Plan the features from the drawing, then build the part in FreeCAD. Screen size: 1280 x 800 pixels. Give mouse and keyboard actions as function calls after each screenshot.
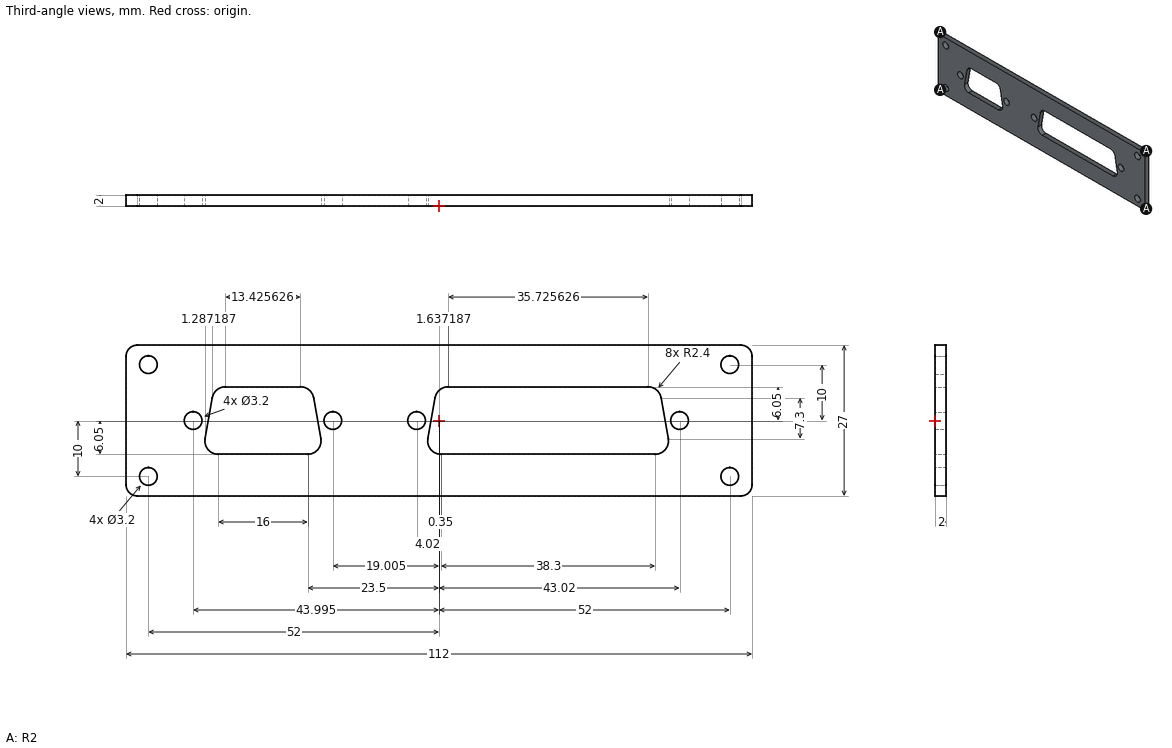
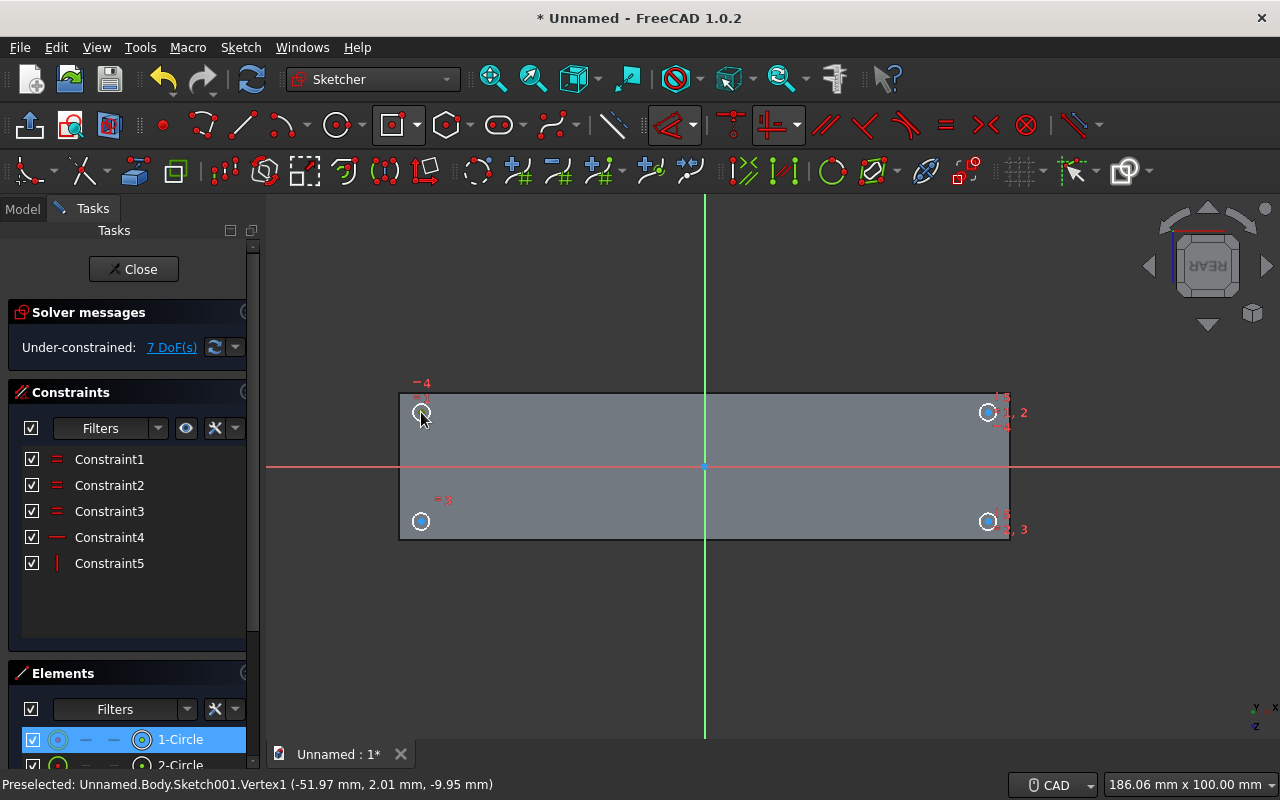
click(421, 522)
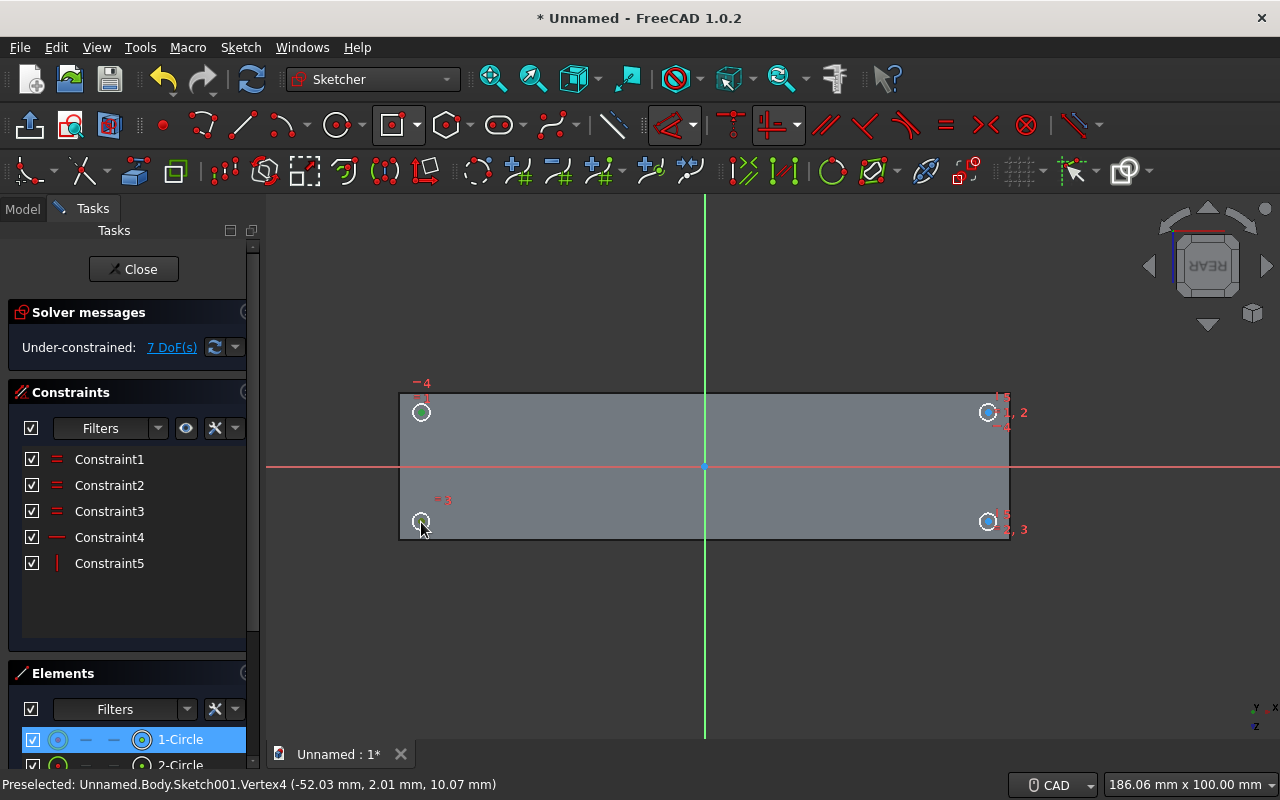
key(v)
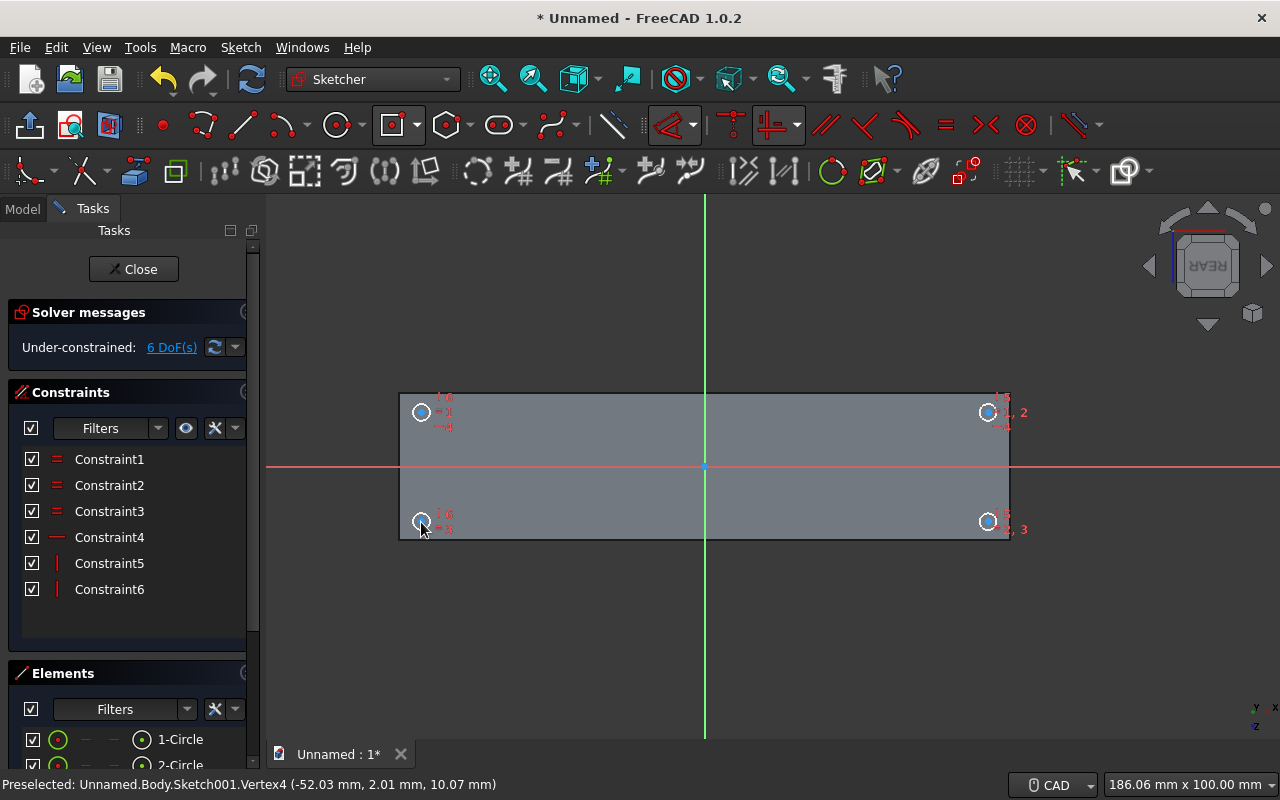
click(988, 522)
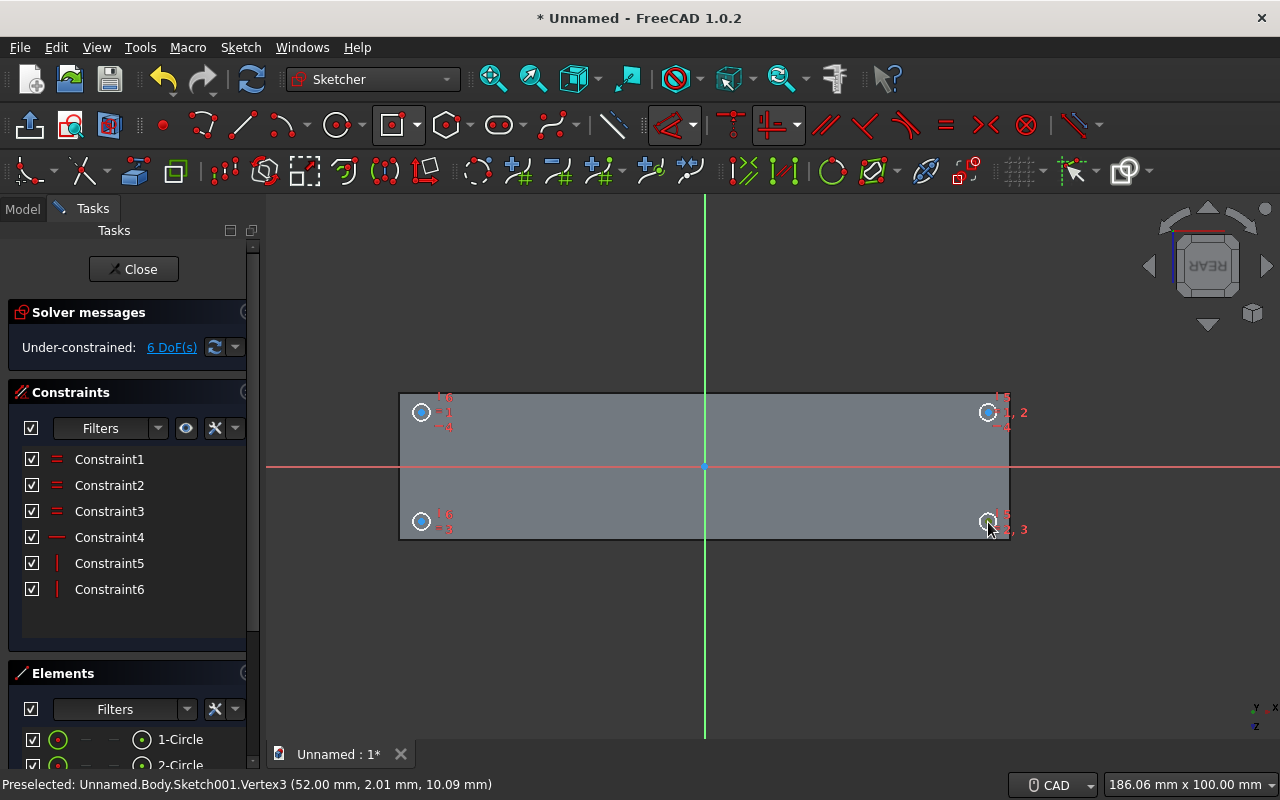
click(421, 522)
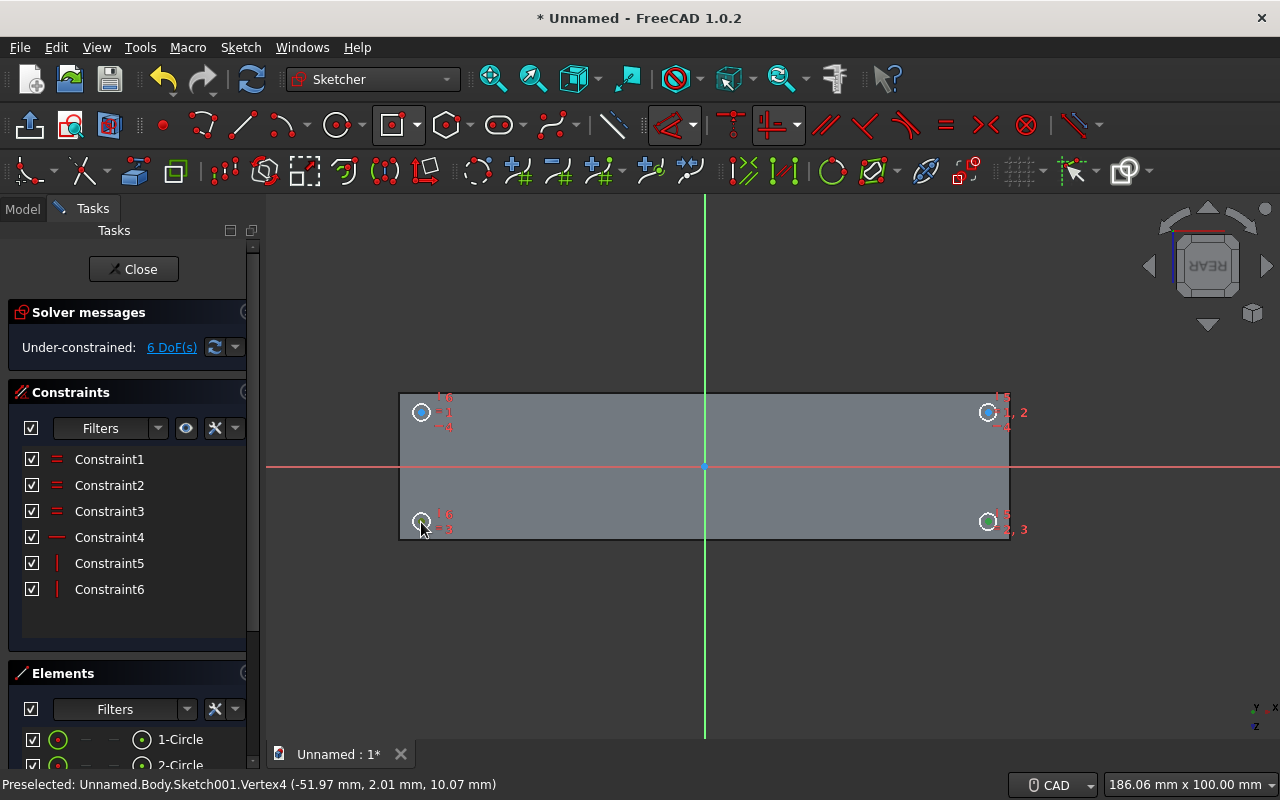
click(800, 126)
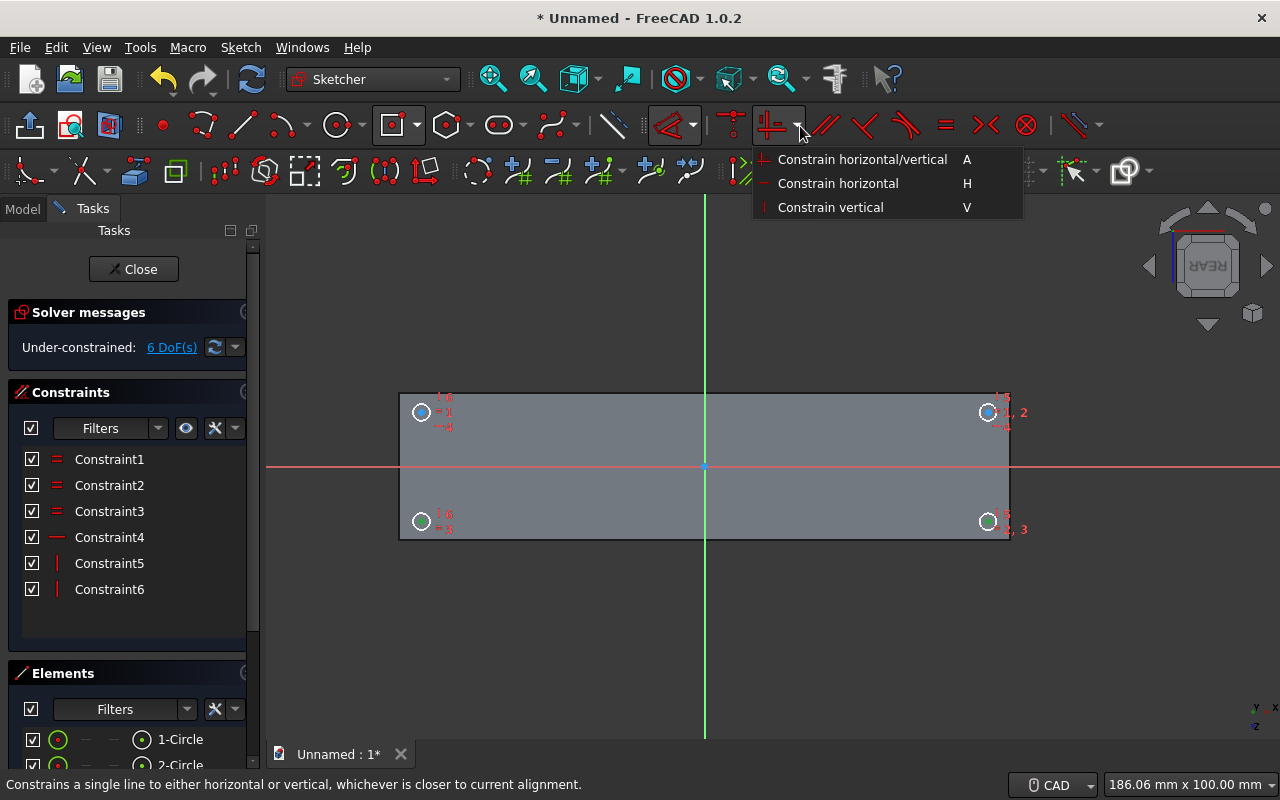
click(888, 183)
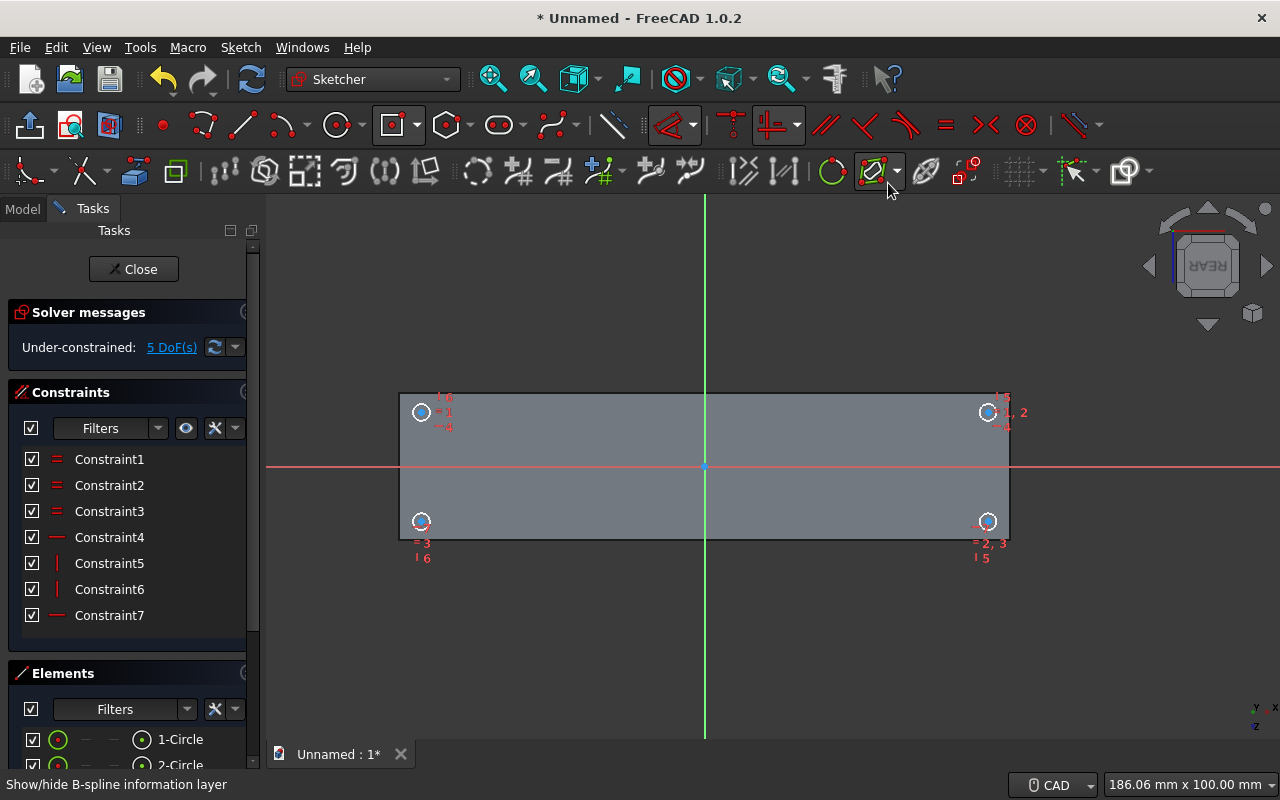
scroll(427, 407, up, 5)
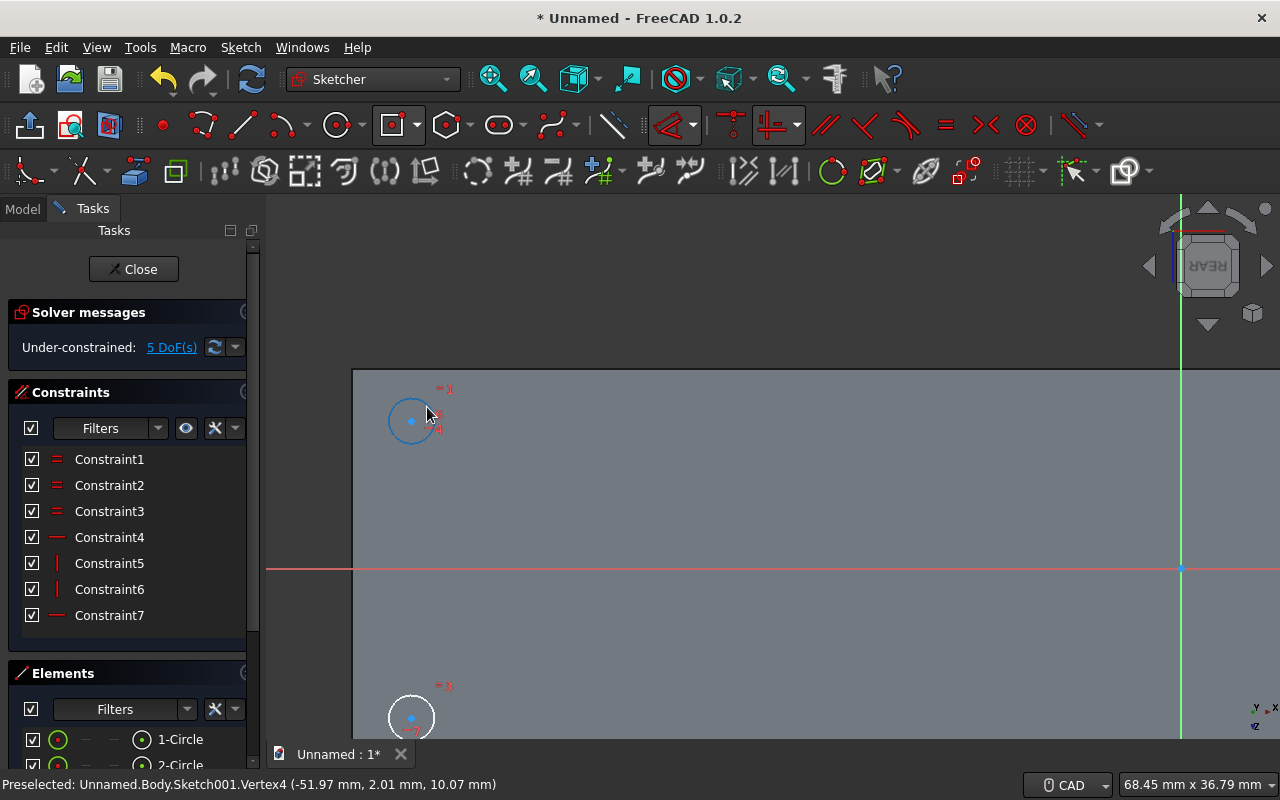
click(428, 405)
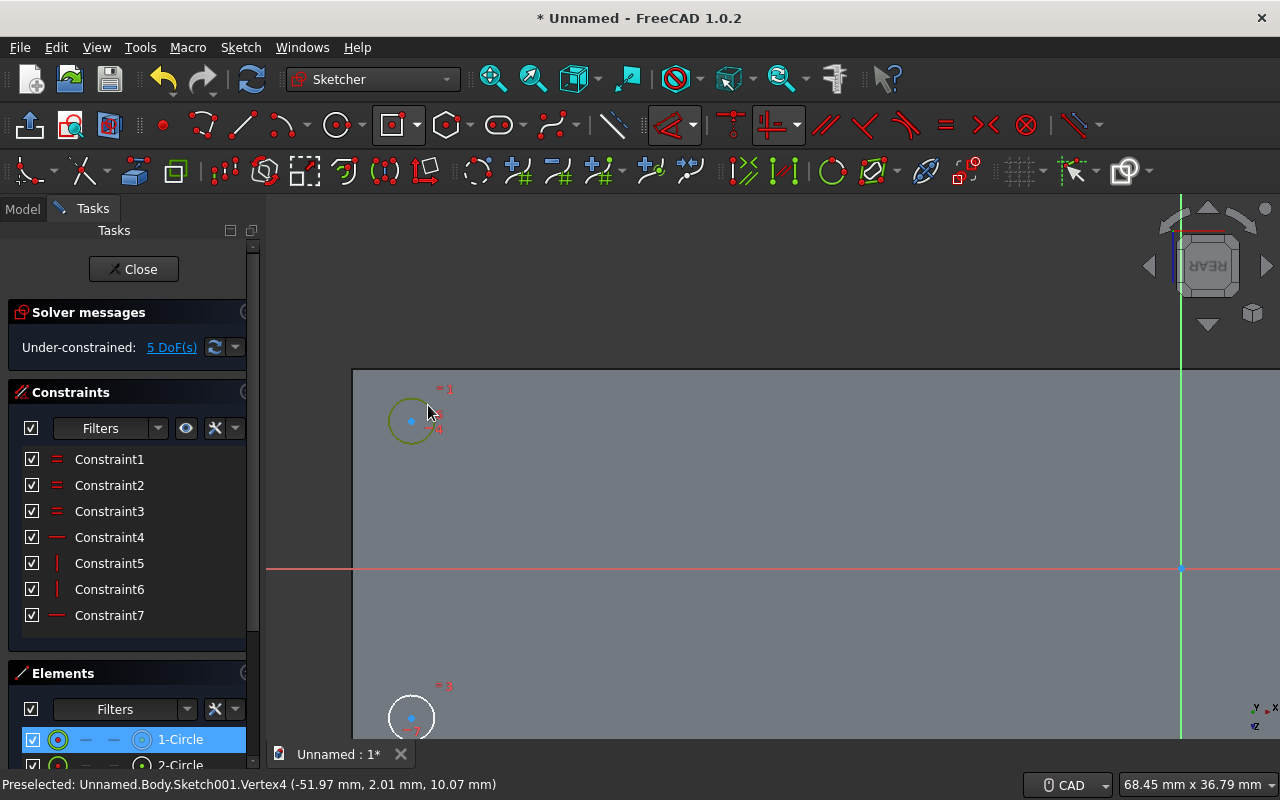
key(k)
key(o)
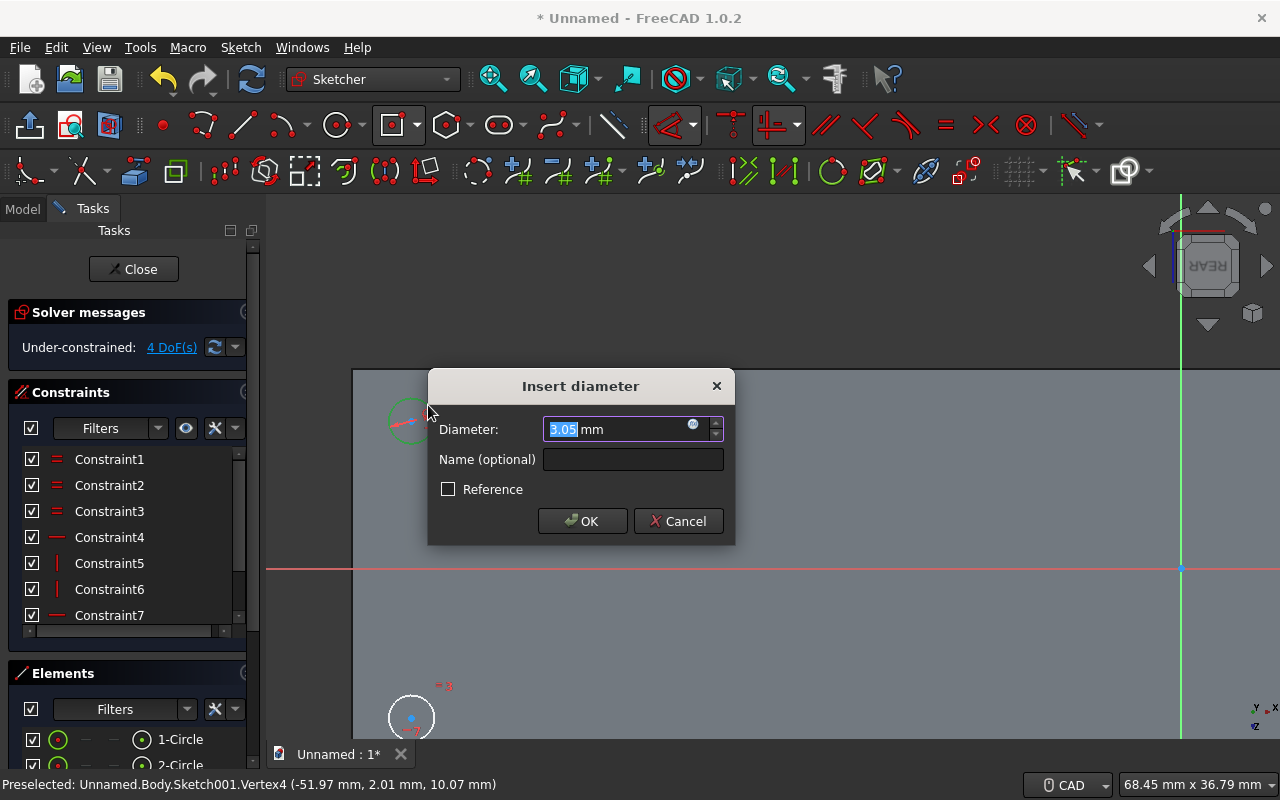
text(3.2)
key(Return)